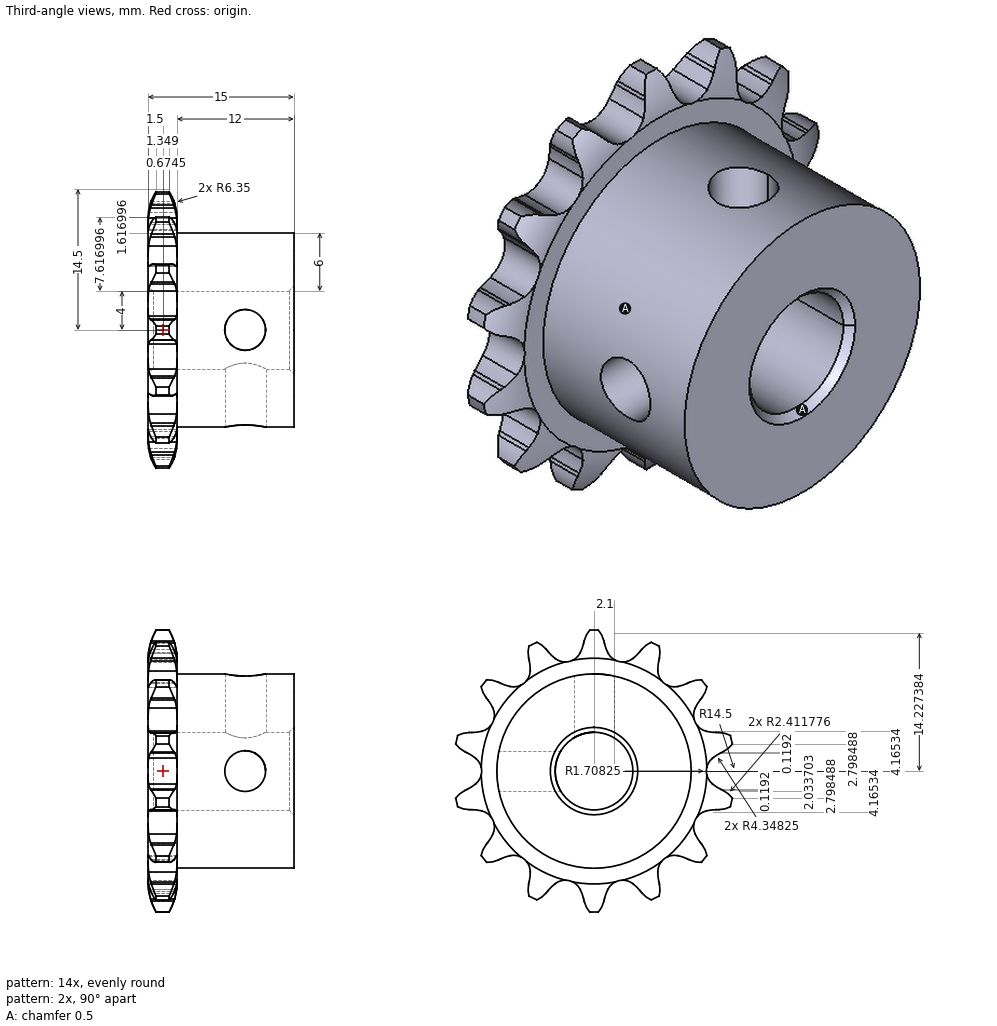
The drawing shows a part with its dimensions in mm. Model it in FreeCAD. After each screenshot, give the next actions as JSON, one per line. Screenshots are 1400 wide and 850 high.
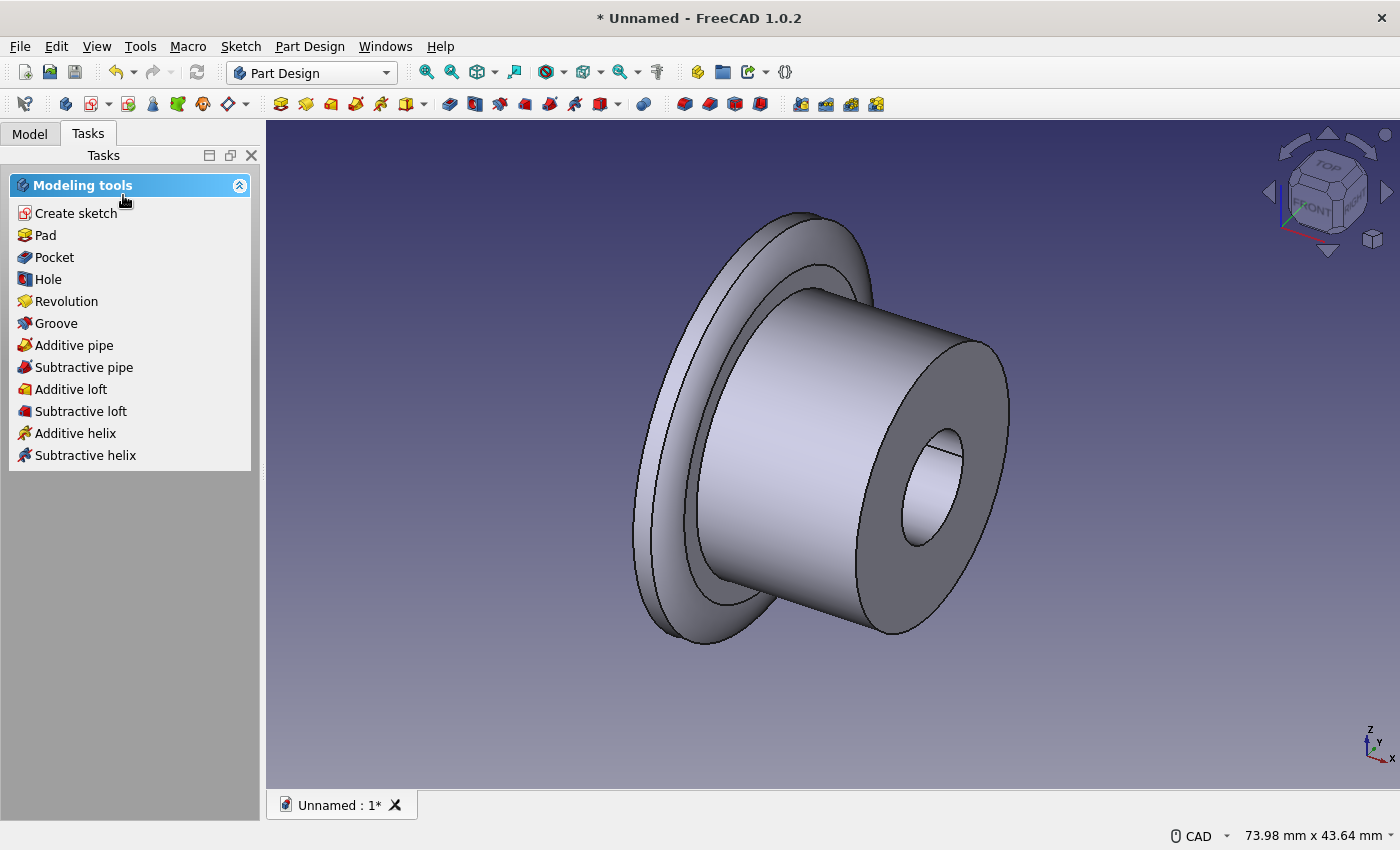
{"action": "left_click", "coordinate": [450, 104]}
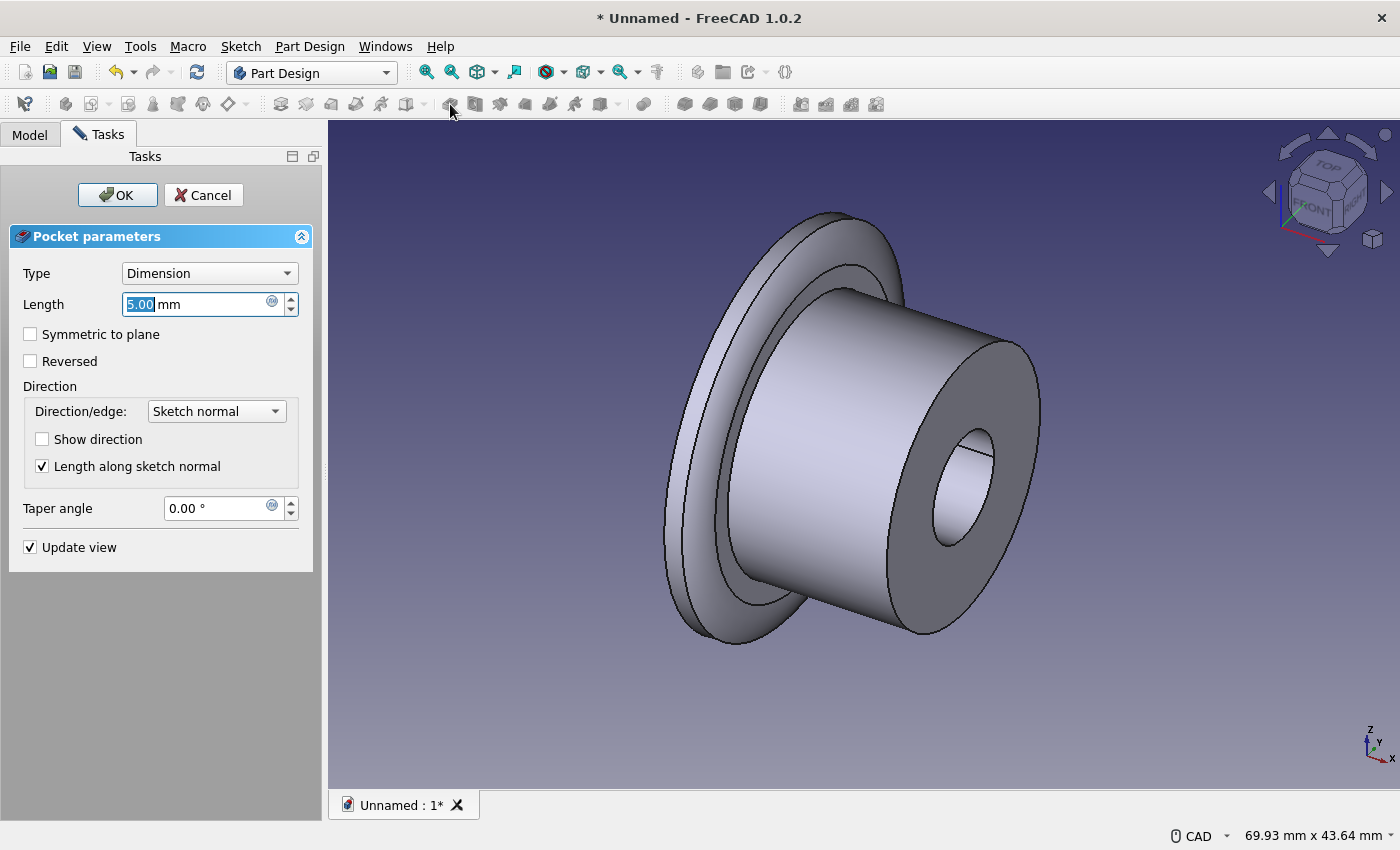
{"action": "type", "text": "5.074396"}
{"action": "key", "text": "Tab"}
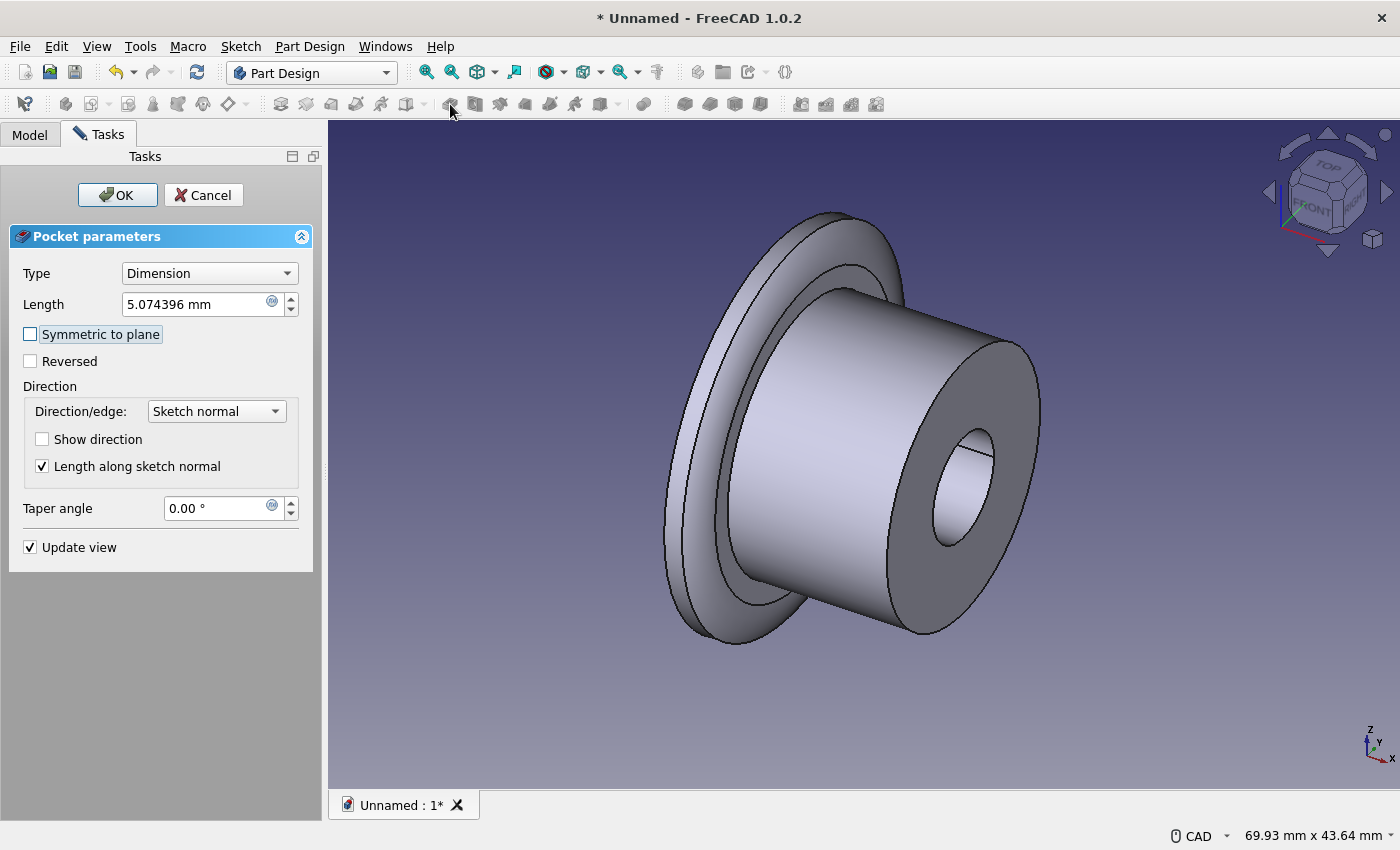
{"action": "left_click", "coordinate": [31, 334]}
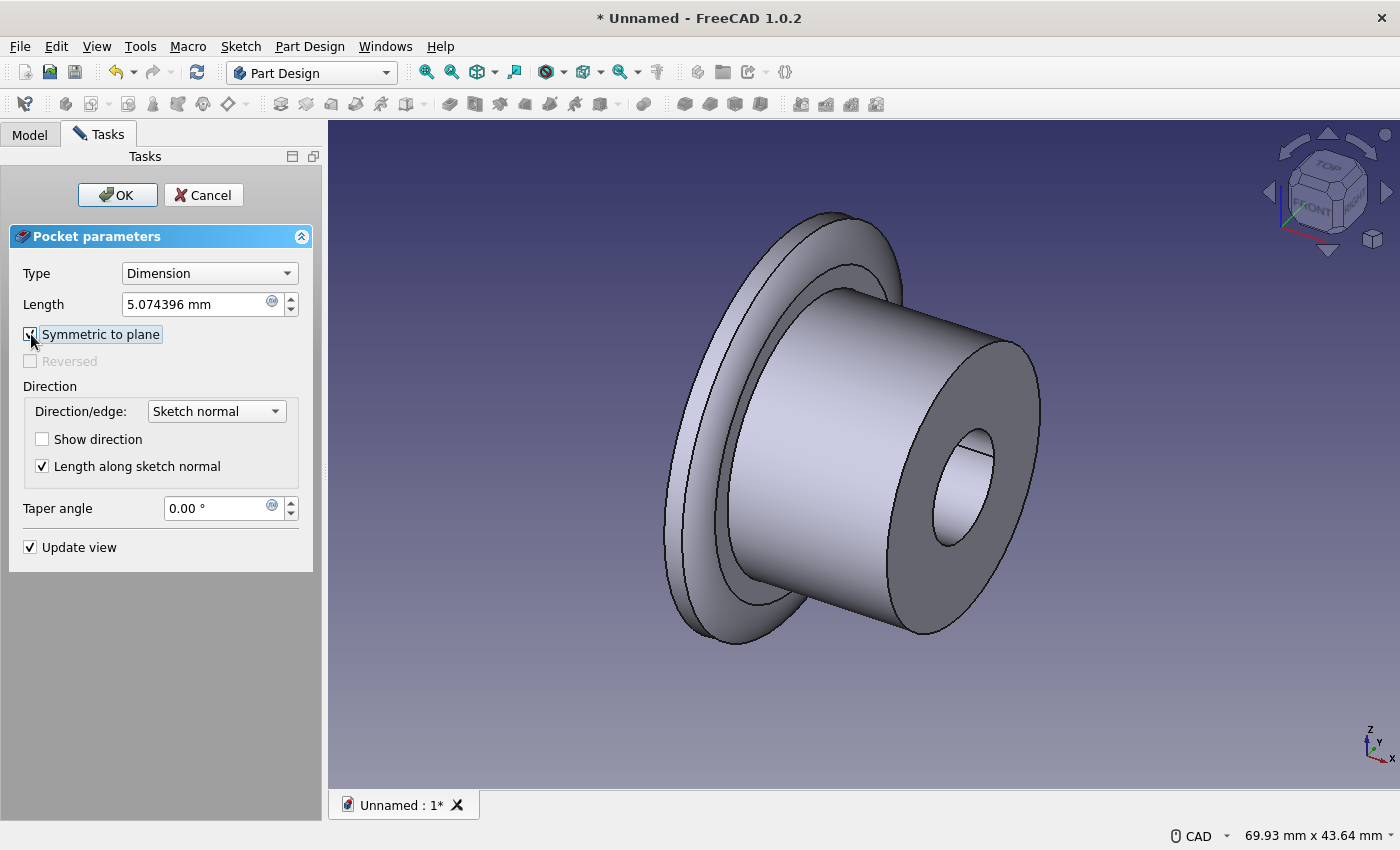
{"action": "left_click", "coordinate": [118, 195]}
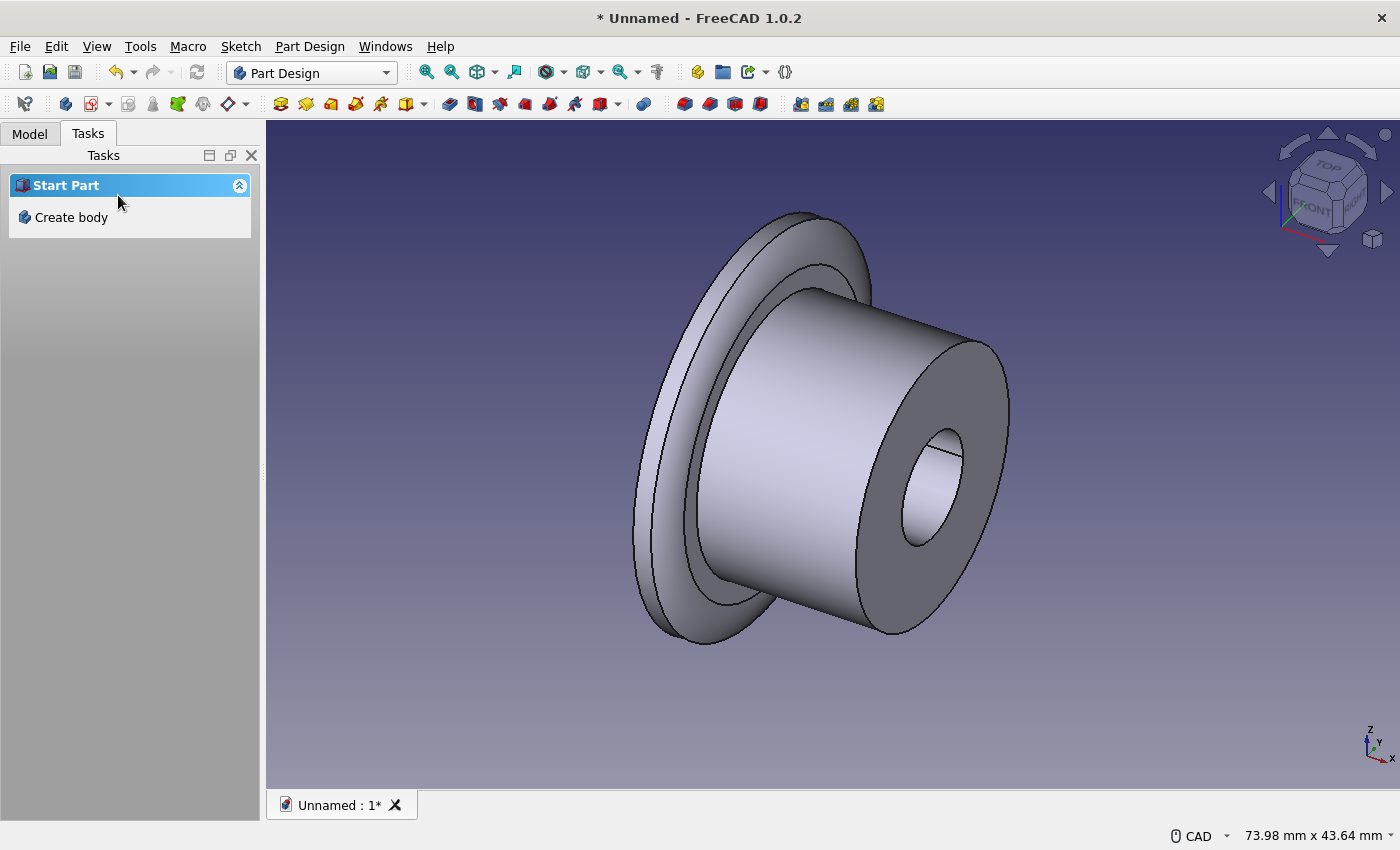
{"action": "left_click", "coordinate": [30, 134]}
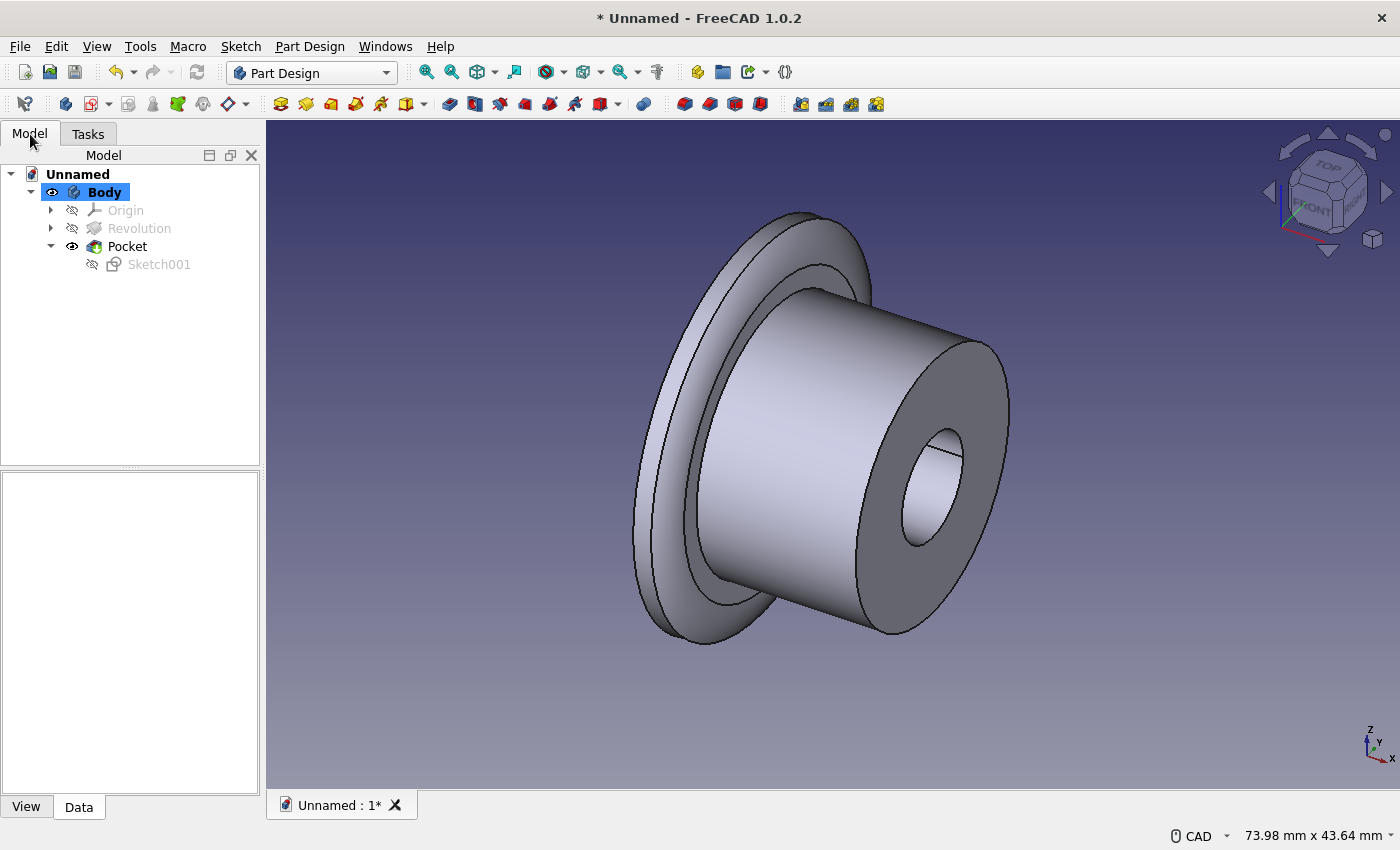
{"action": "left_click", "coordinate": [117, 246]}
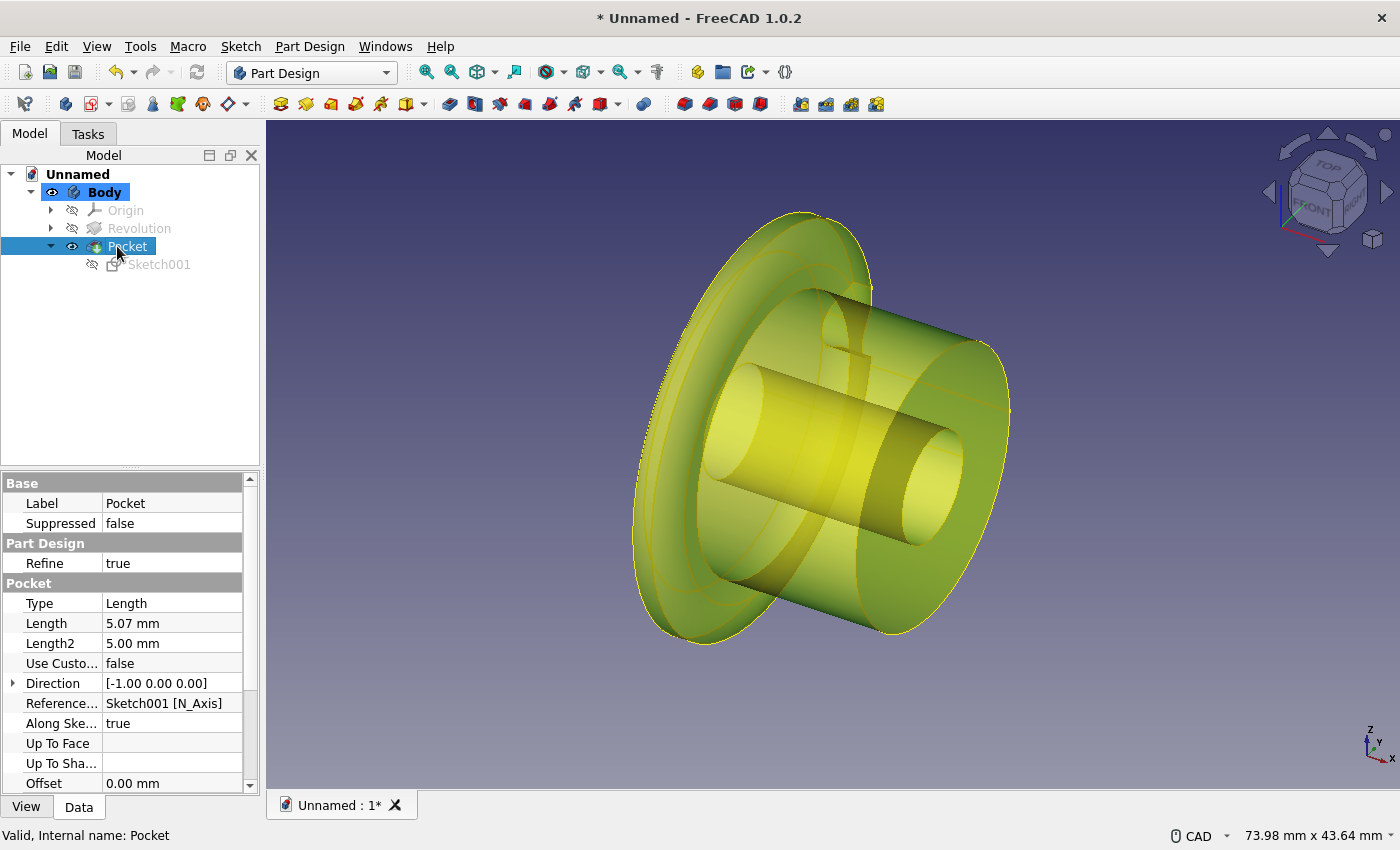
{"action": "left_click", "coordinate": [851, 104]}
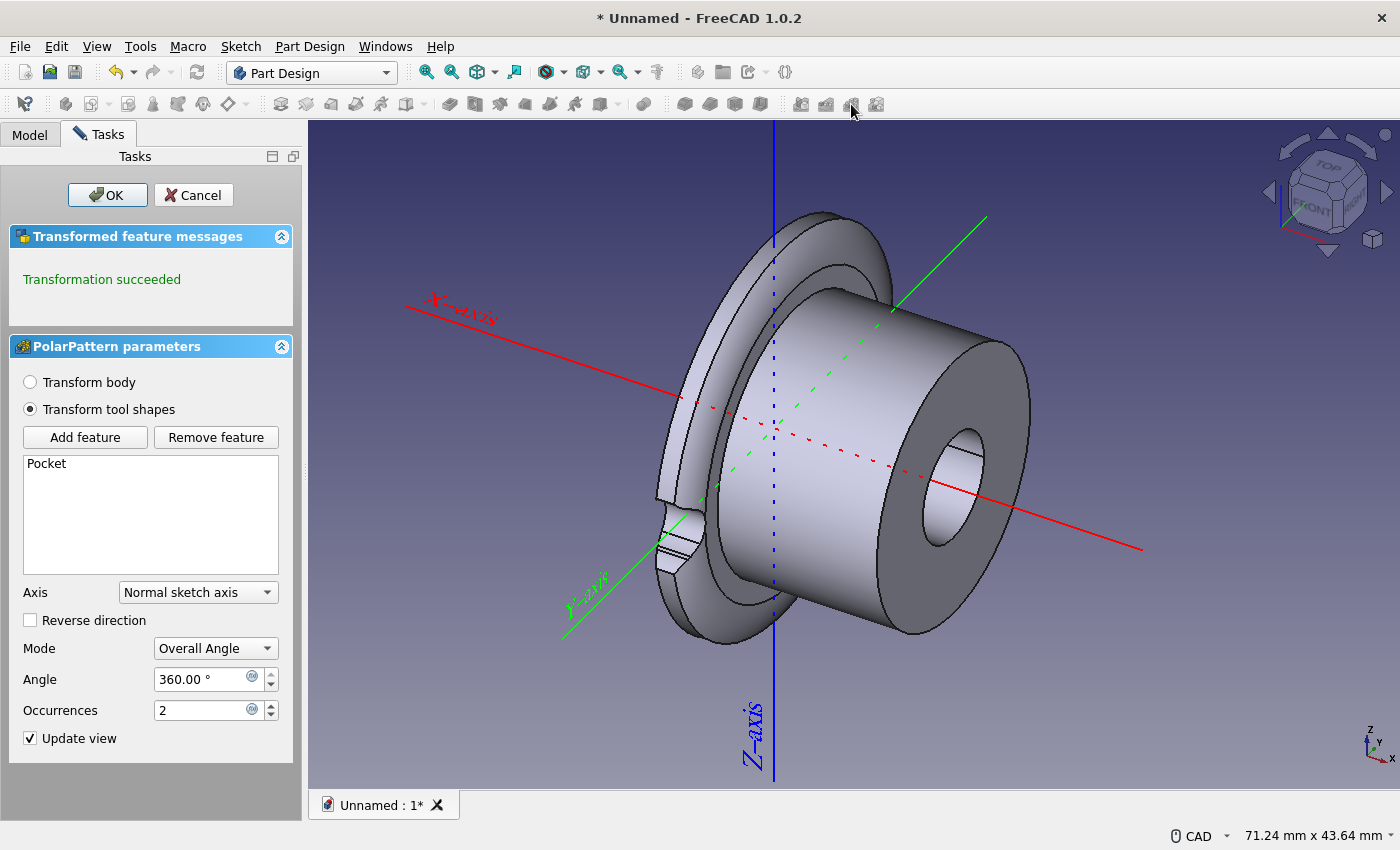
{"action": "left_click", "coordinate": [199, 592]}